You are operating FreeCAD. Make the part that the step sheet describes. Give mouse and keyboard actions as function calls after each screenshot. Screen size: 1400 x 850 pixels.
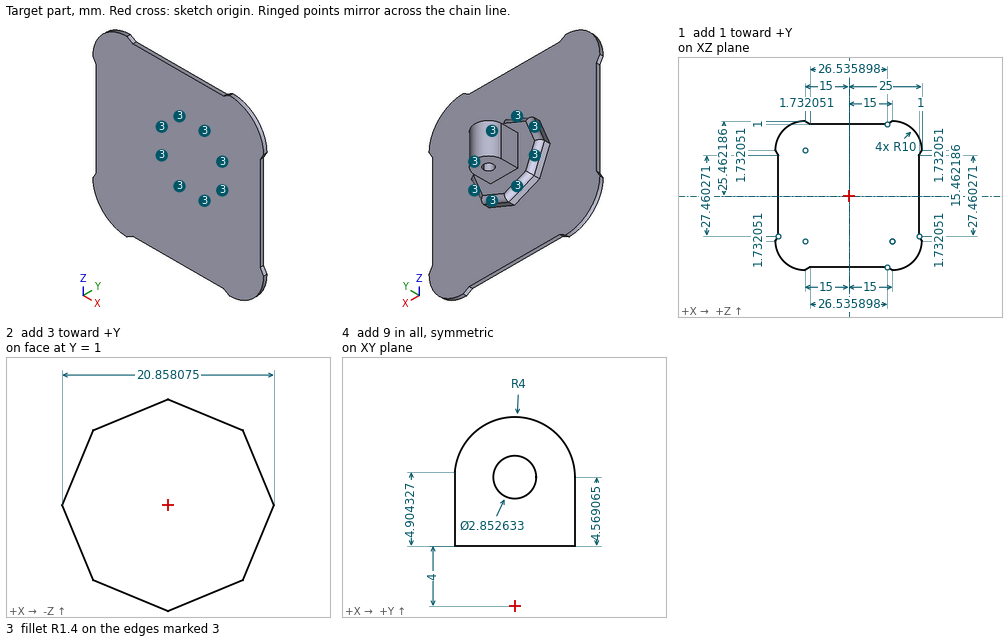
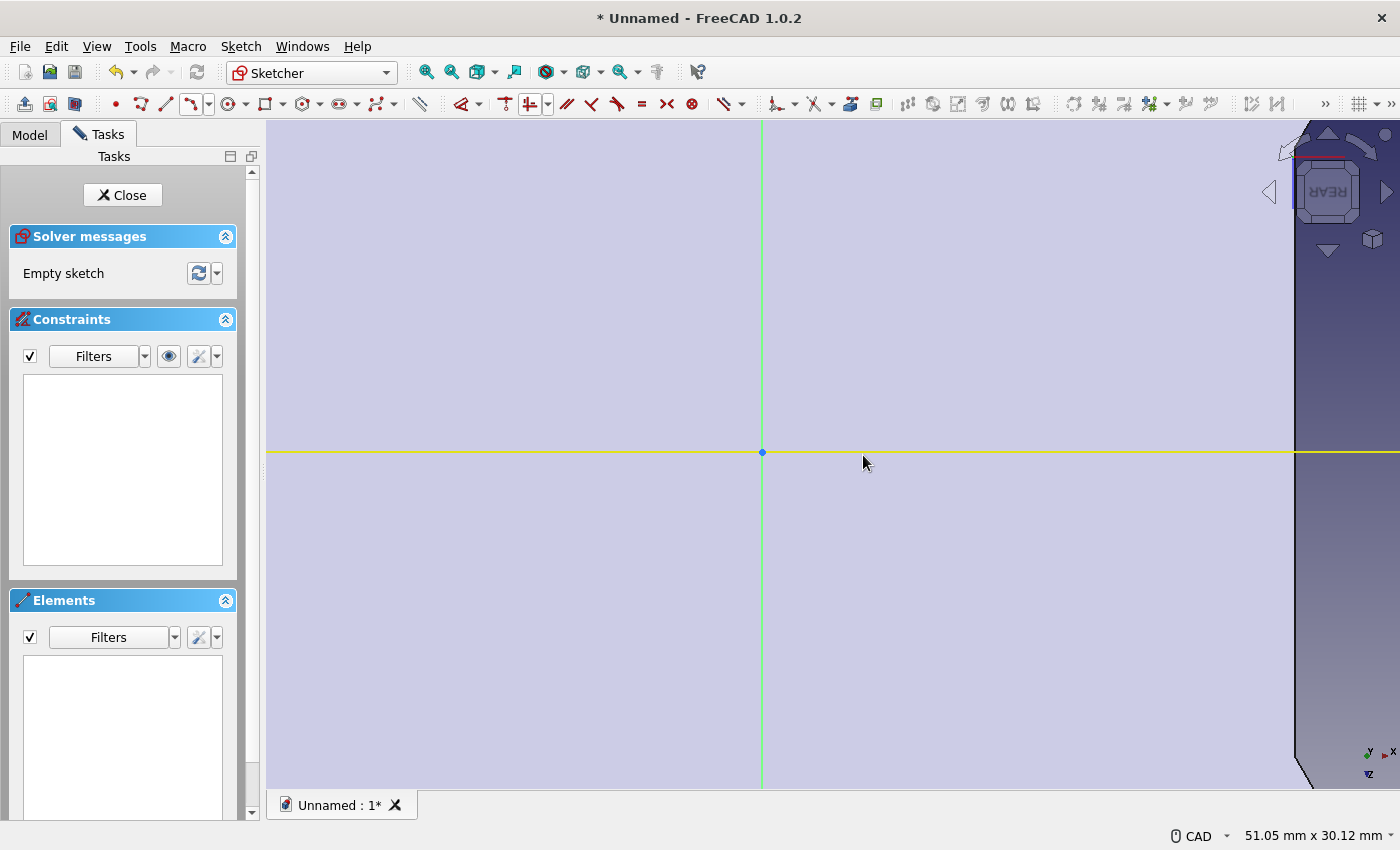
key(g)
key(p)
key(8)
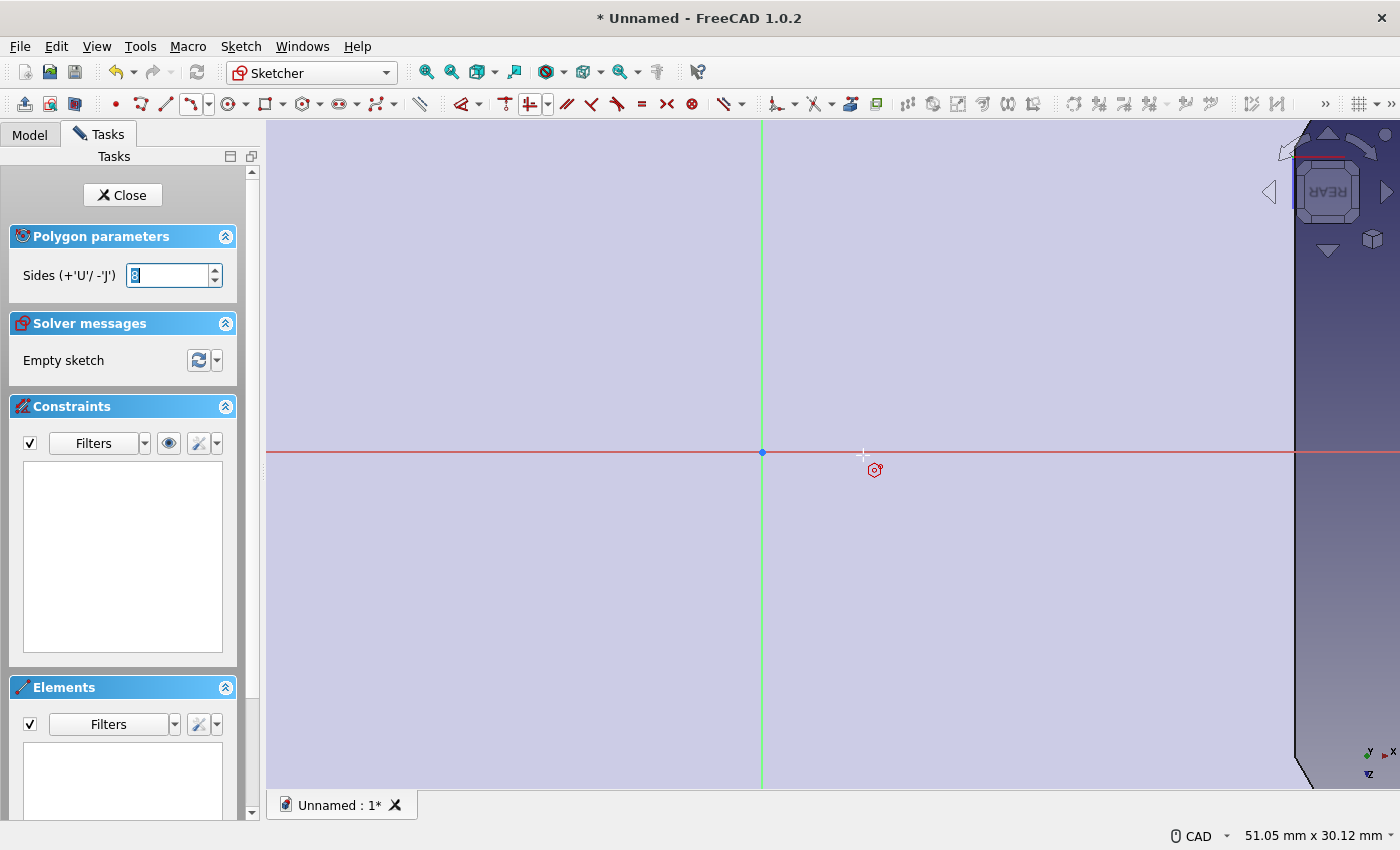
click(762, 452)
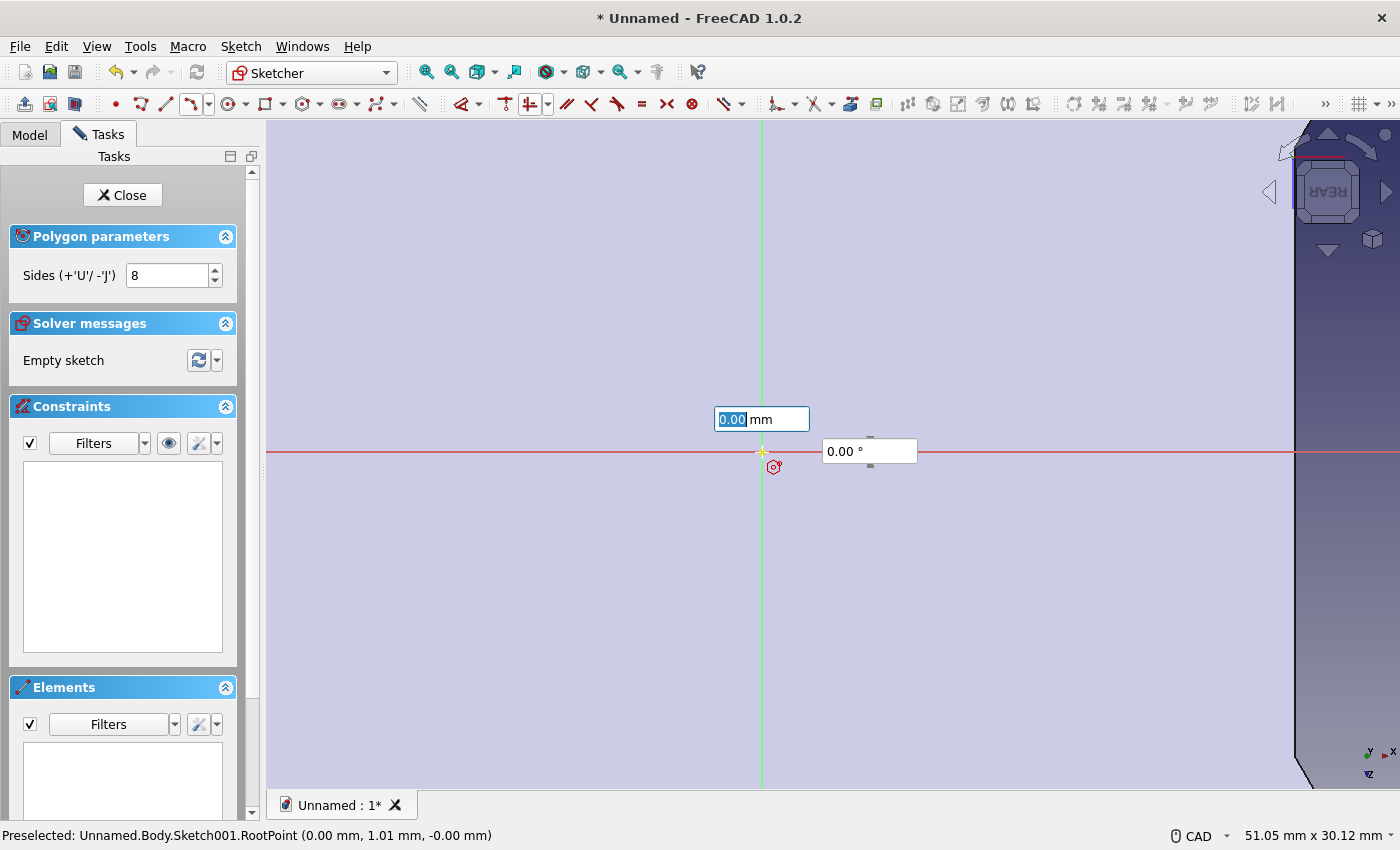
click(762, 684)
right_click(762, 684)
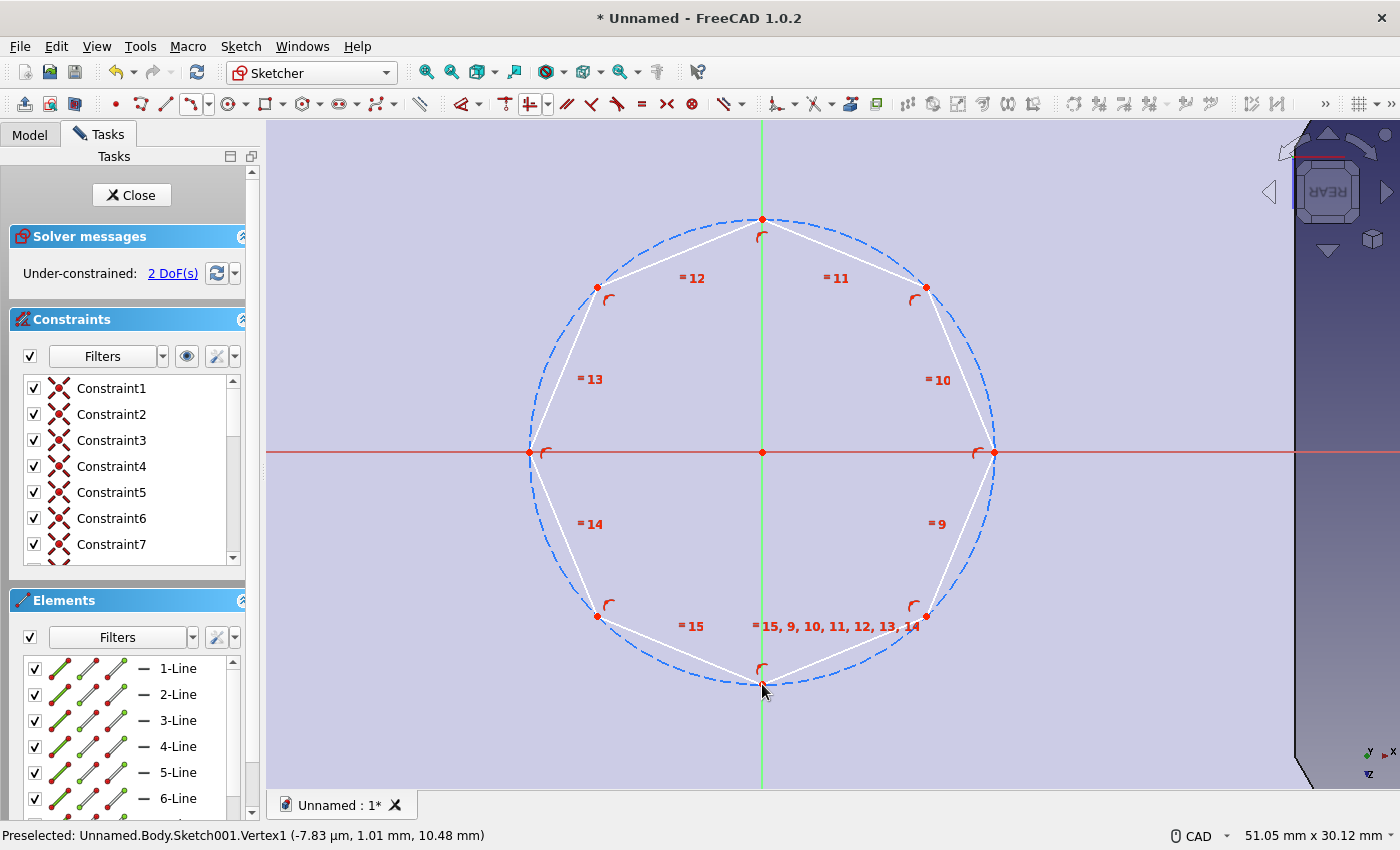
click(762, 685)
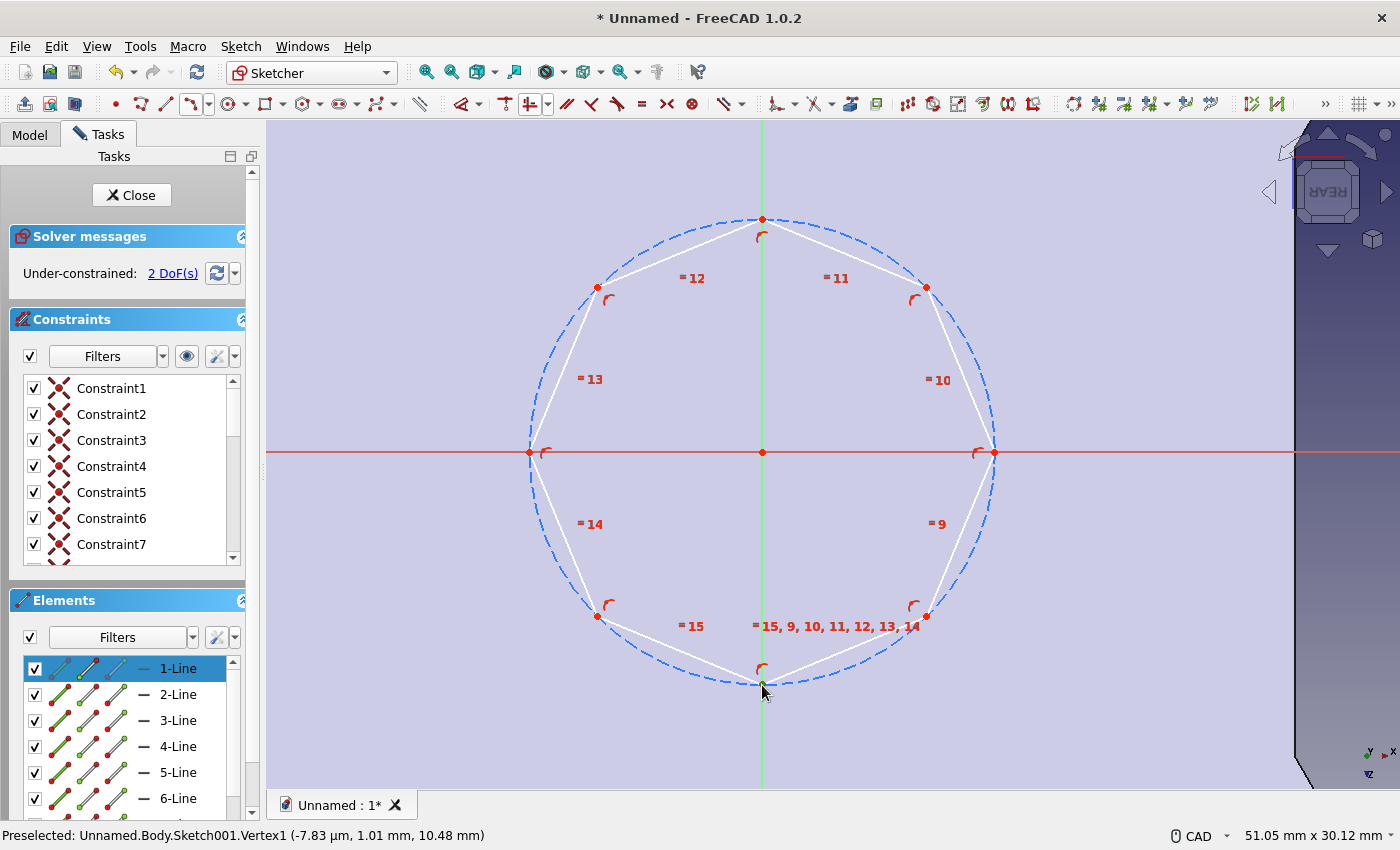
click(762, 717)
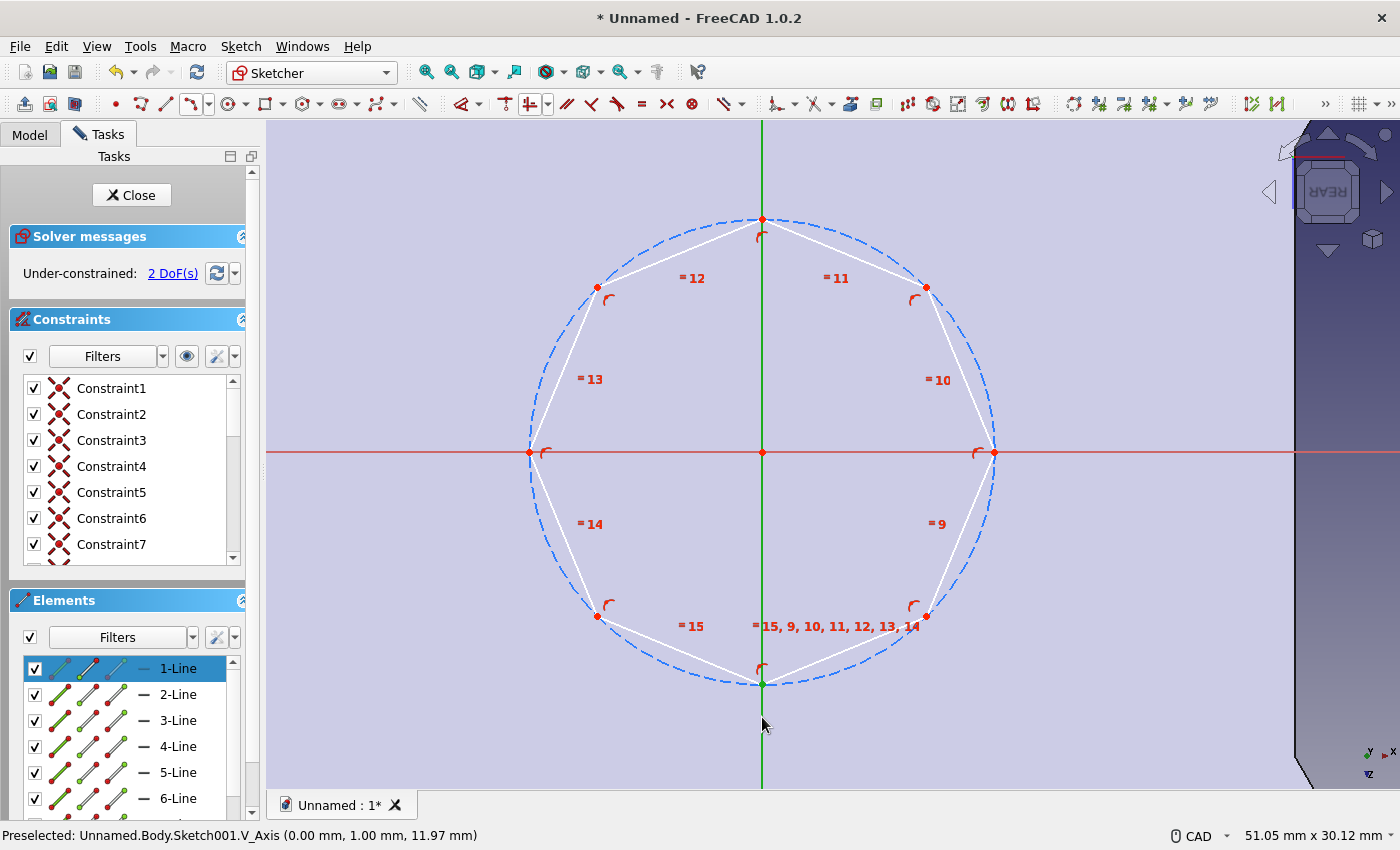
click(505, 104)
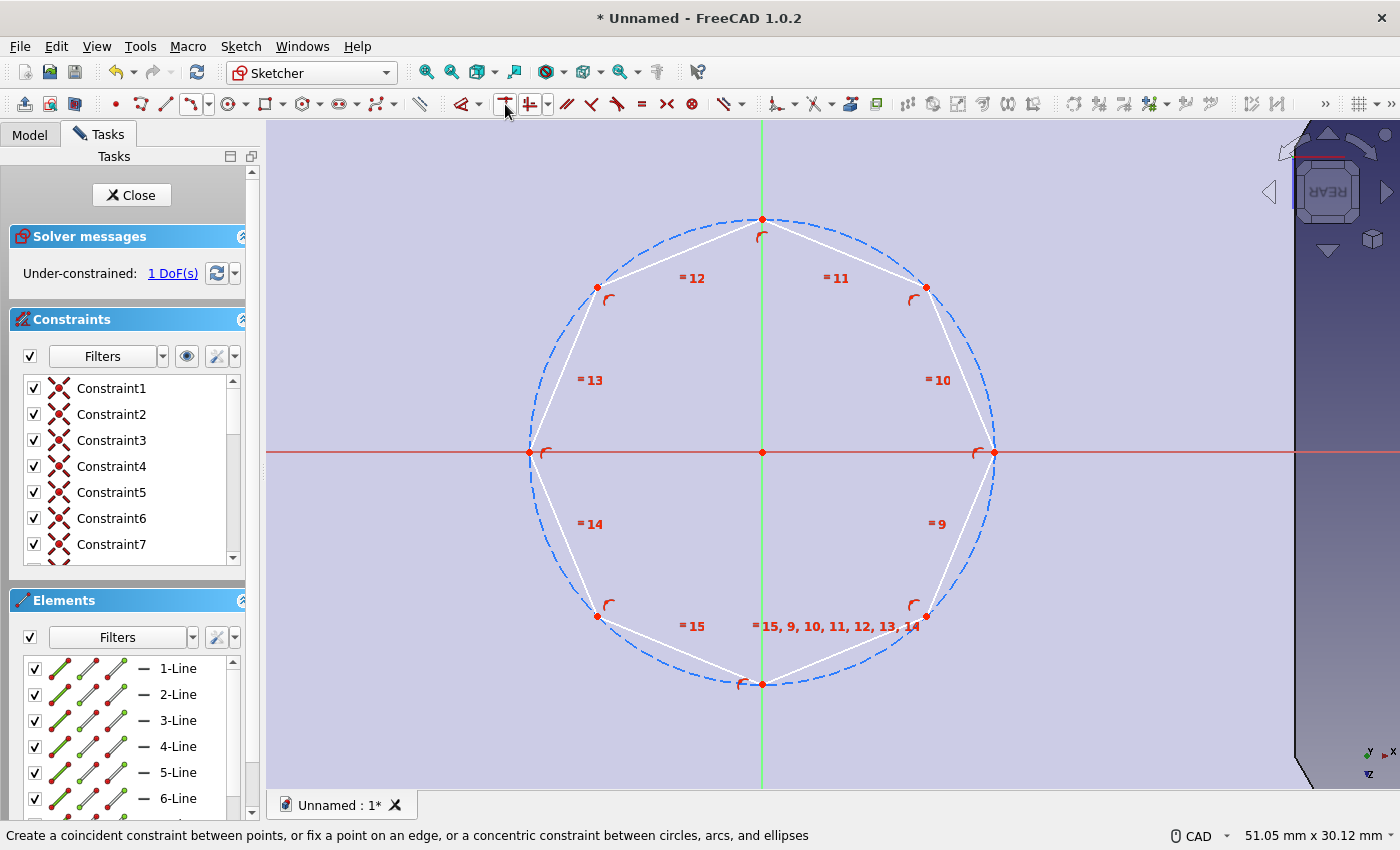
click(460, 104)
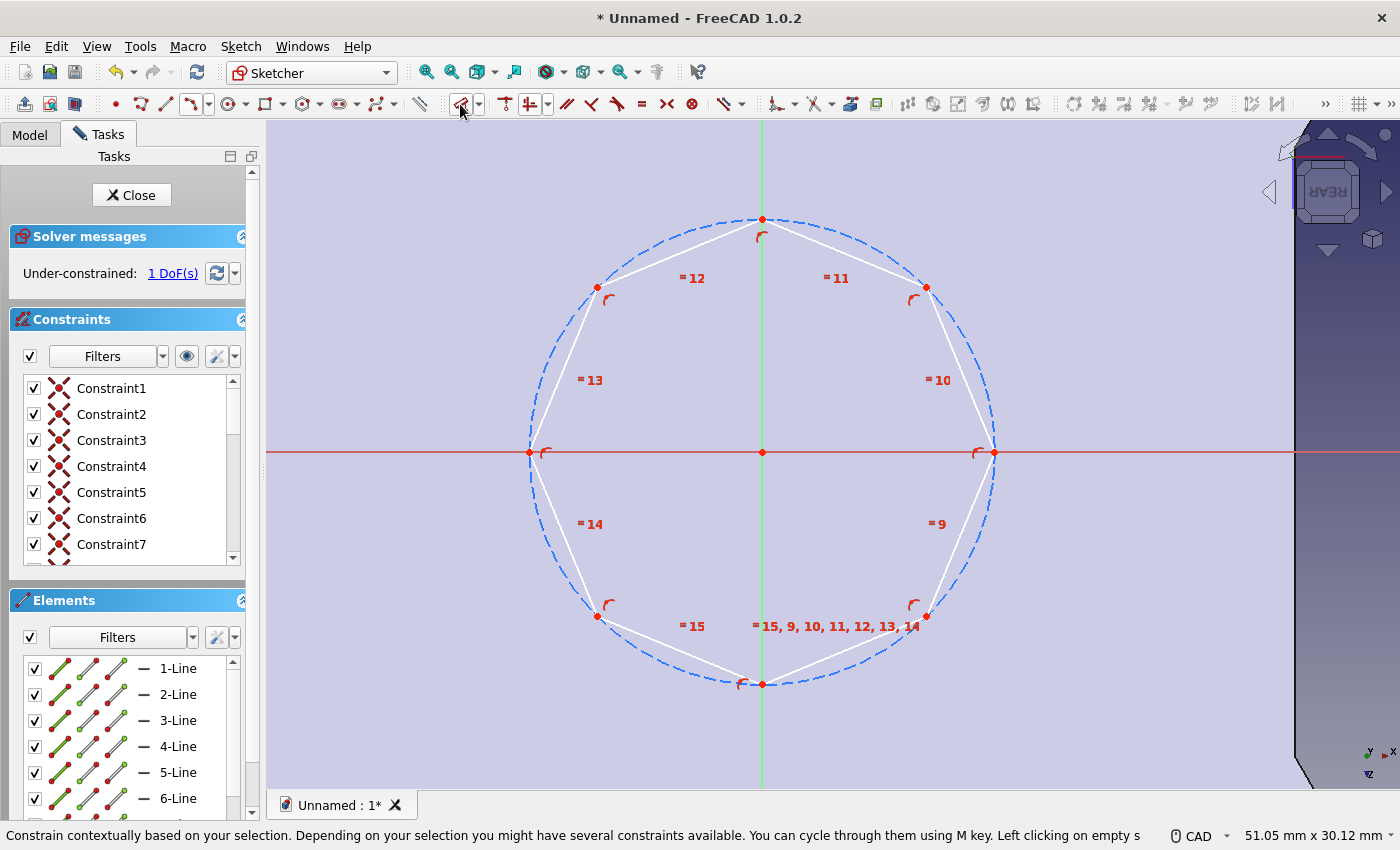
click(529, 452)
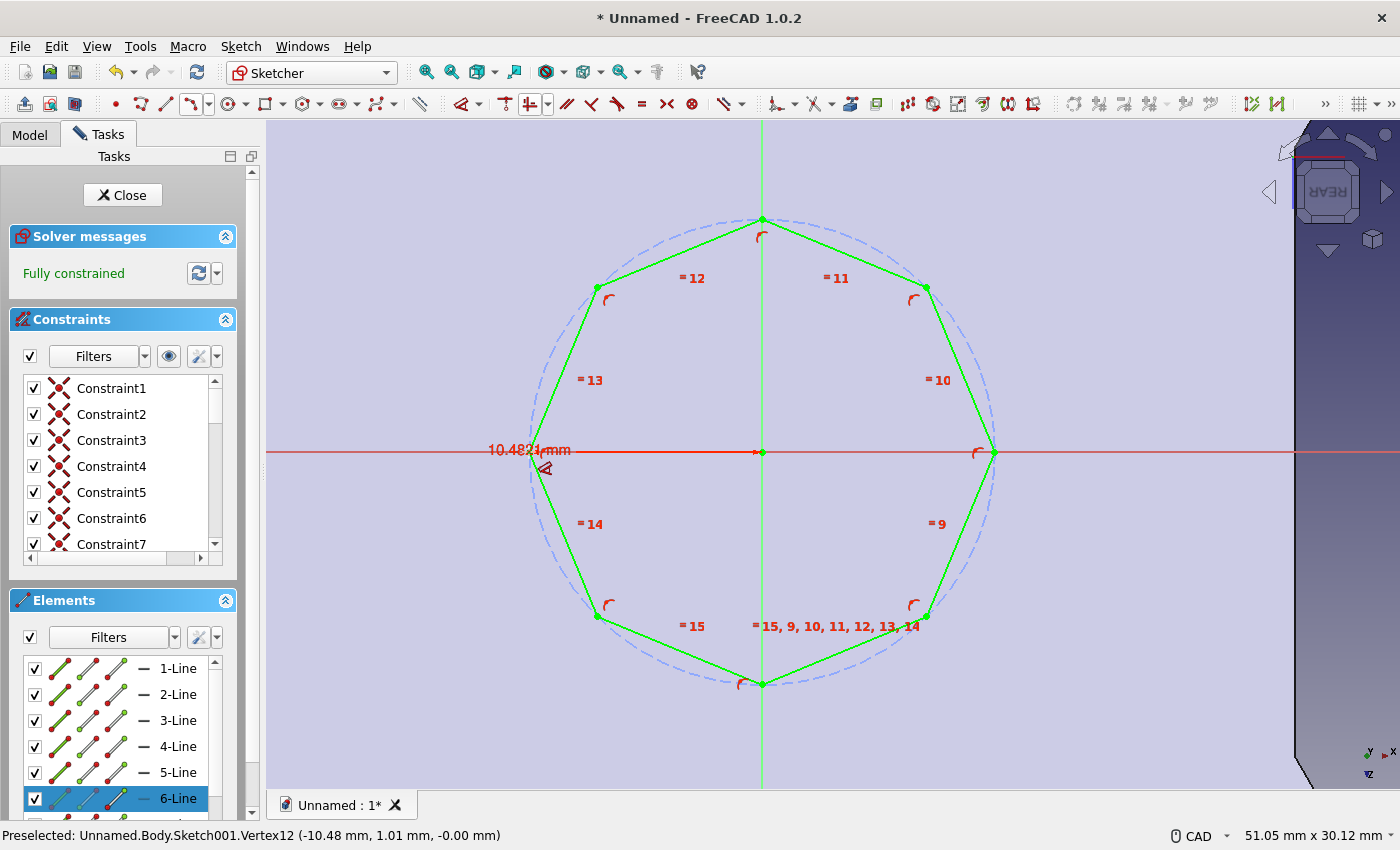
click(995, 452)
click(655, 486)